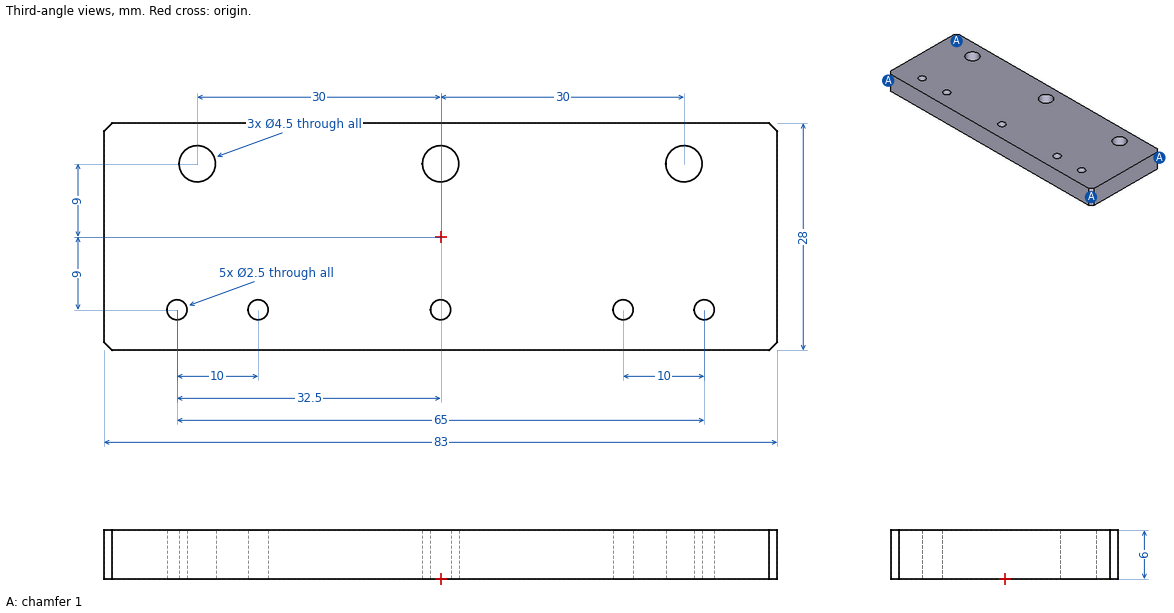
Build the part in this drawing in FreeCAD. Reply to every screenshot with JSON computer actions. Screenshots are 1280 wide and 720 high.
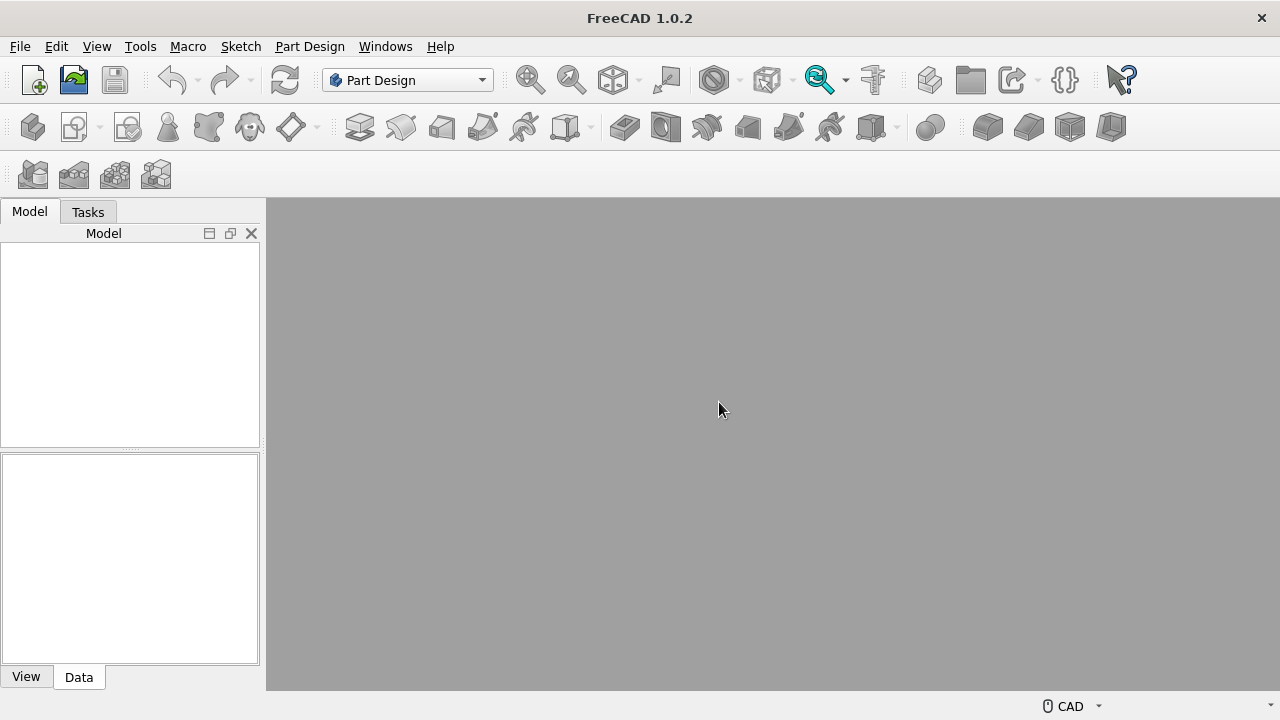
{"action": "left_click", "coordinate": [33, 80]}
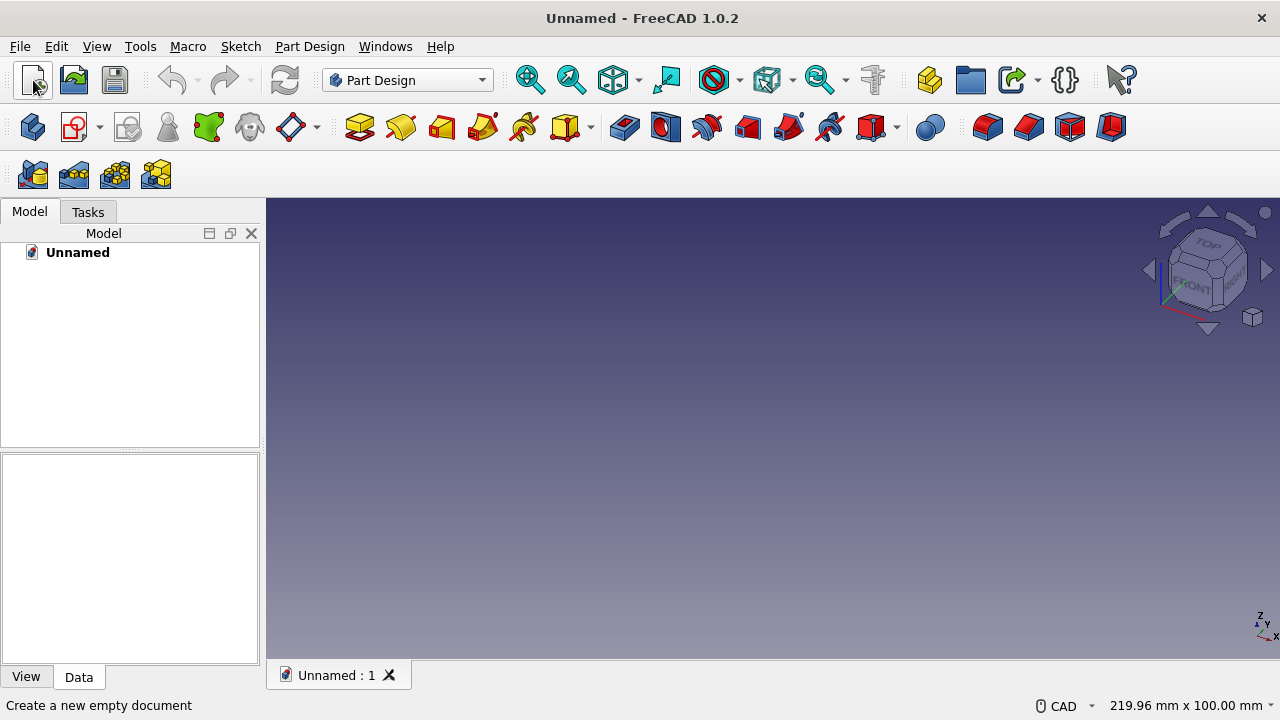
{"action": "left_click", "coordinate": [74, 128]}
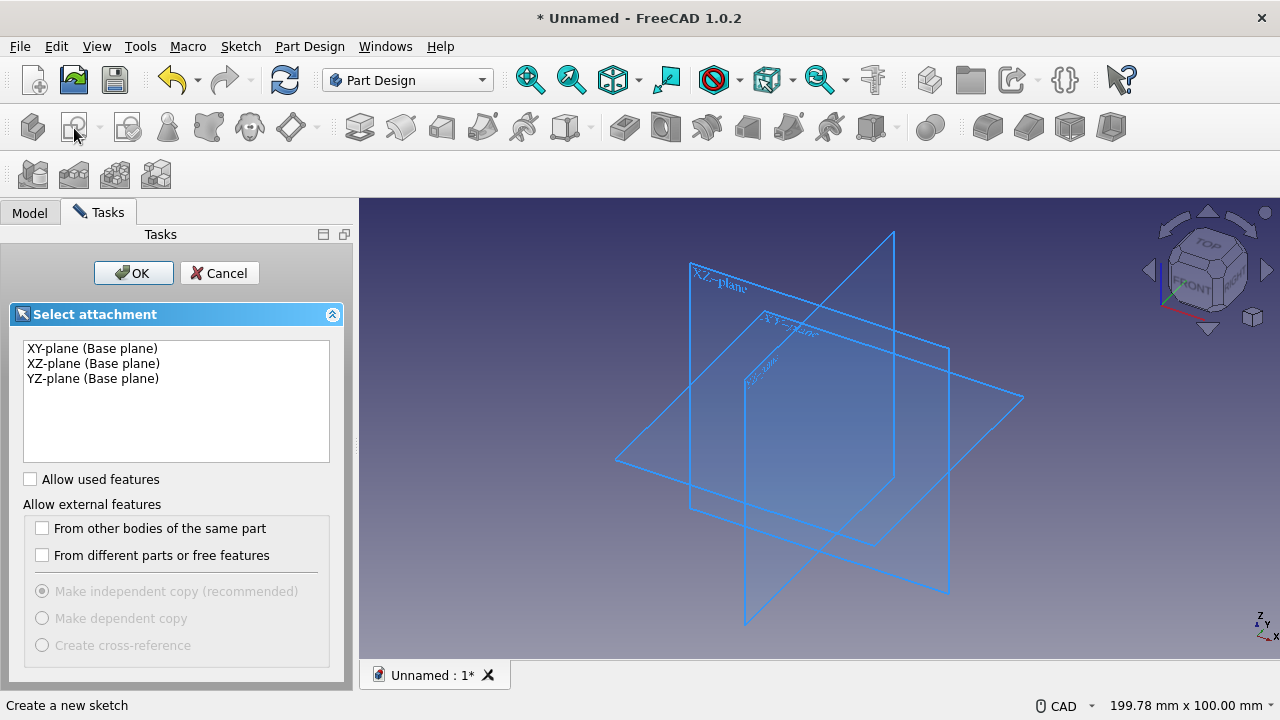
{"action": "left_click", "coordinate": [84, 348]}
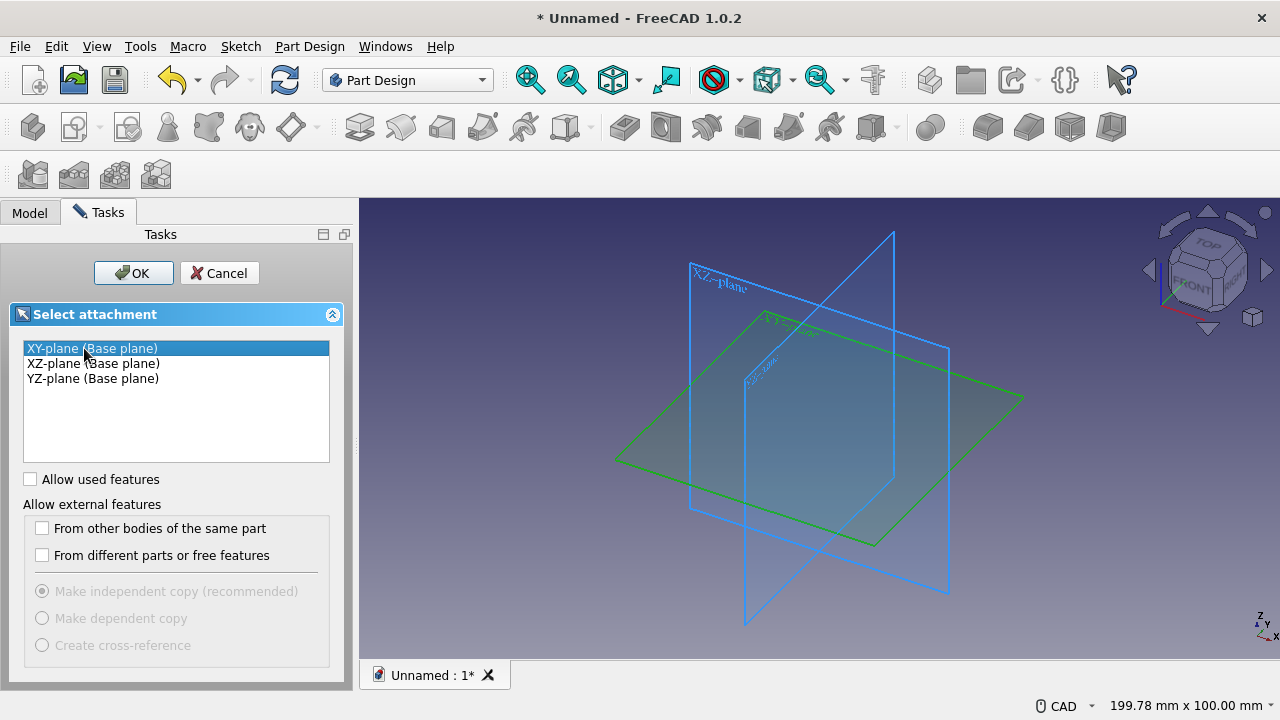
{"action": "left_click", "coordinate": [134, 273]}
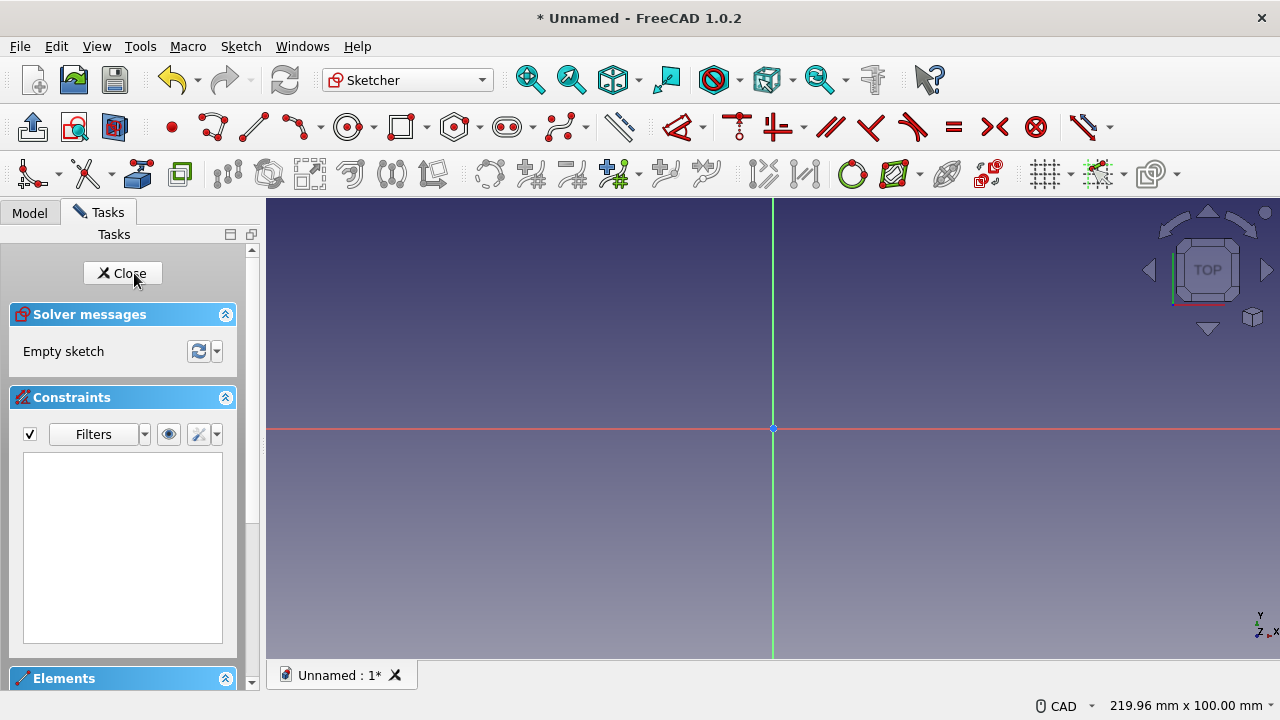
{"action": "scroll", "coordinate": [912, 428], "scroll_direction": "up", "scroll_amount": 2}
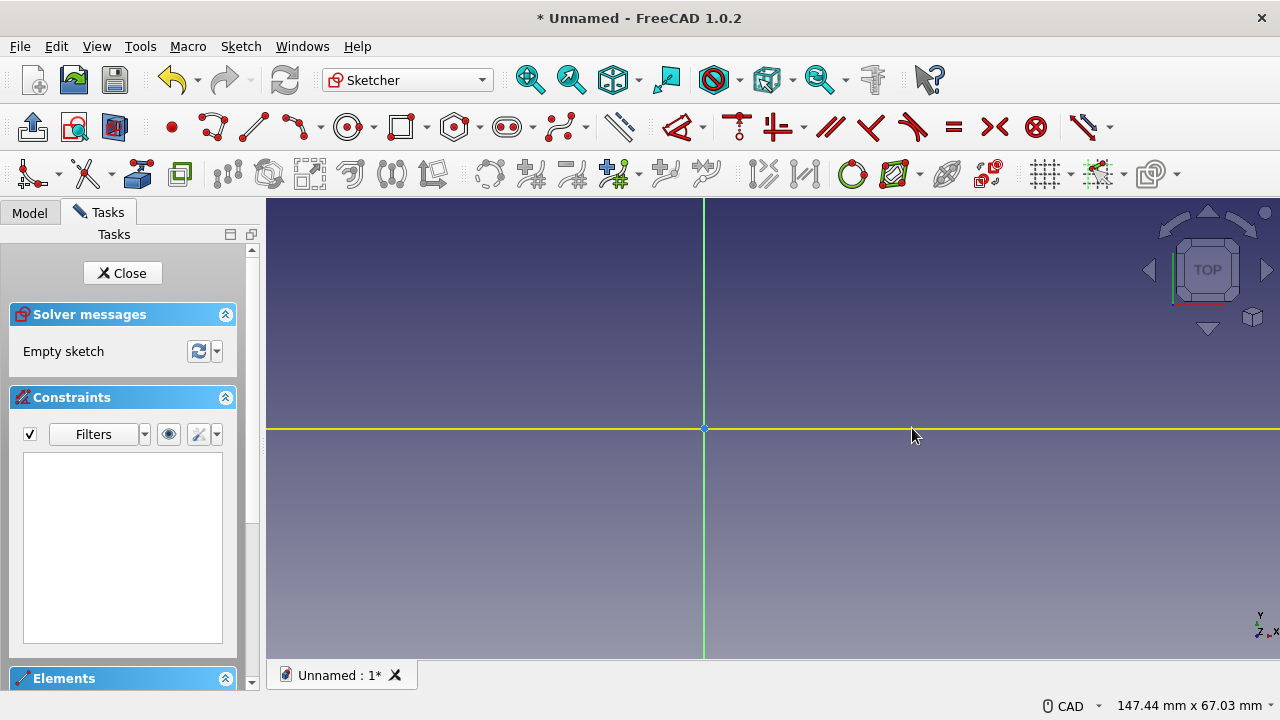
{"action": "key", "text": "g v"}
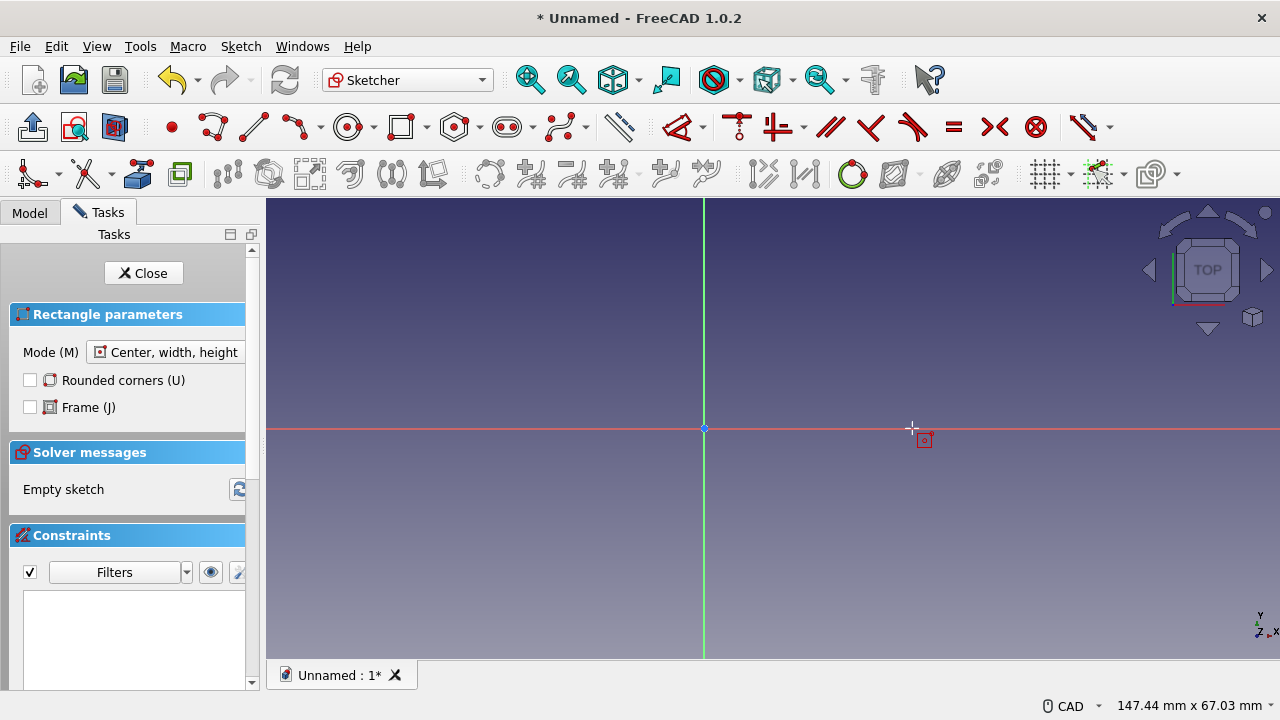
{"action": "left_click", "coordinate": [704, 428]}
{"action": "left_click", "coordinate": [990, 332]}
{"action": "key", "text": "Escape"}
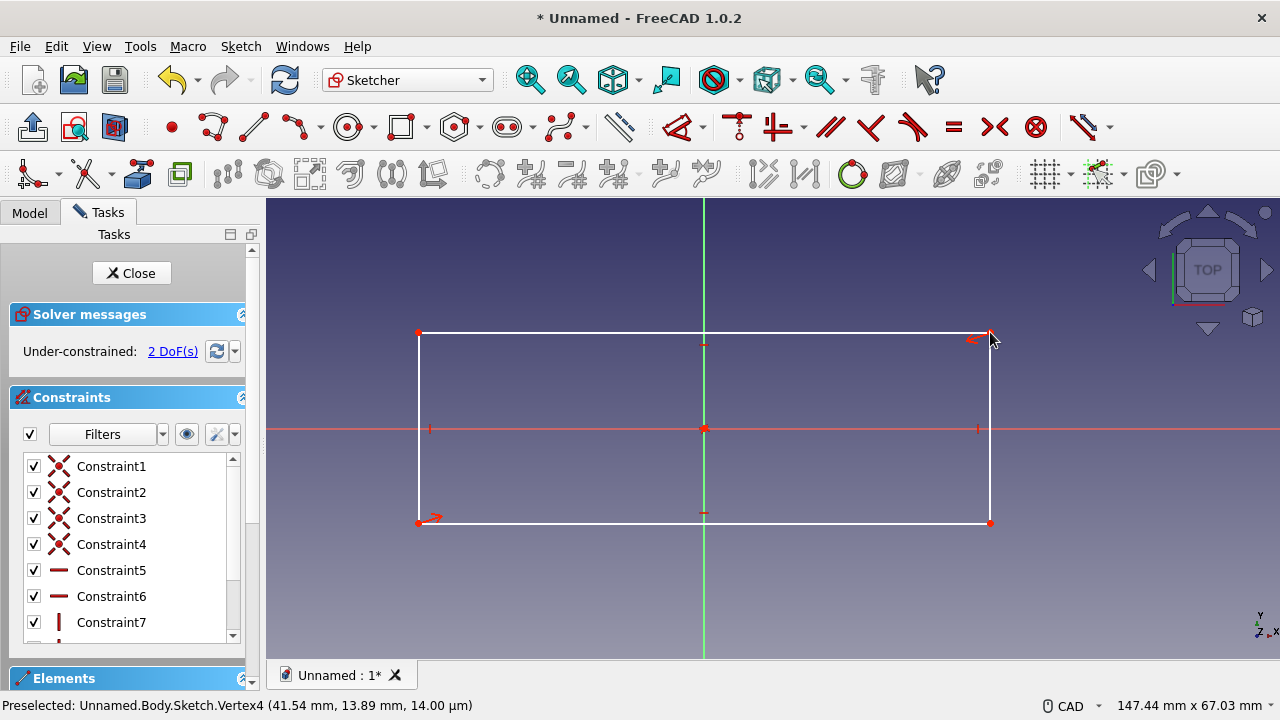
{"action": "left_click", "coordinate": [676, 128]}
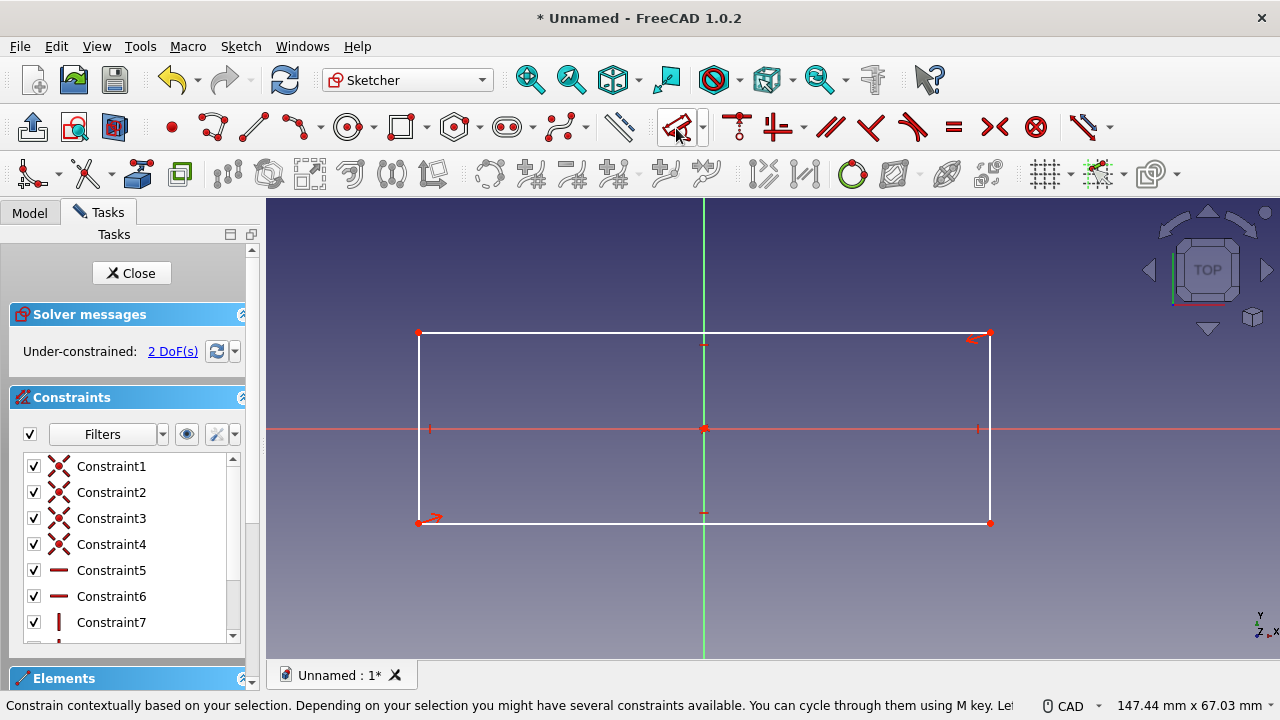
{"action": "left_click", "coordinate": [590, 524]}
{"action": "left_click", "coordinate": [573, 558]}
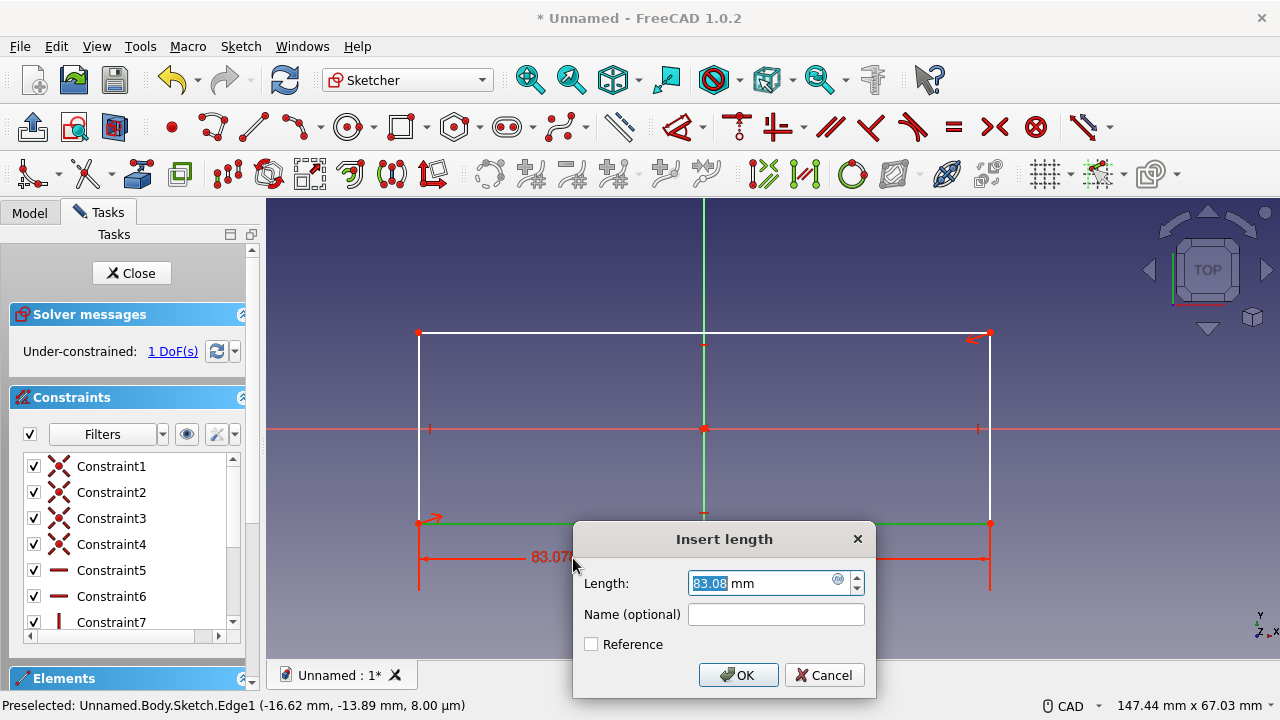
{"action": "type", "text": "83"}
{"action": "key", "text": "Return"}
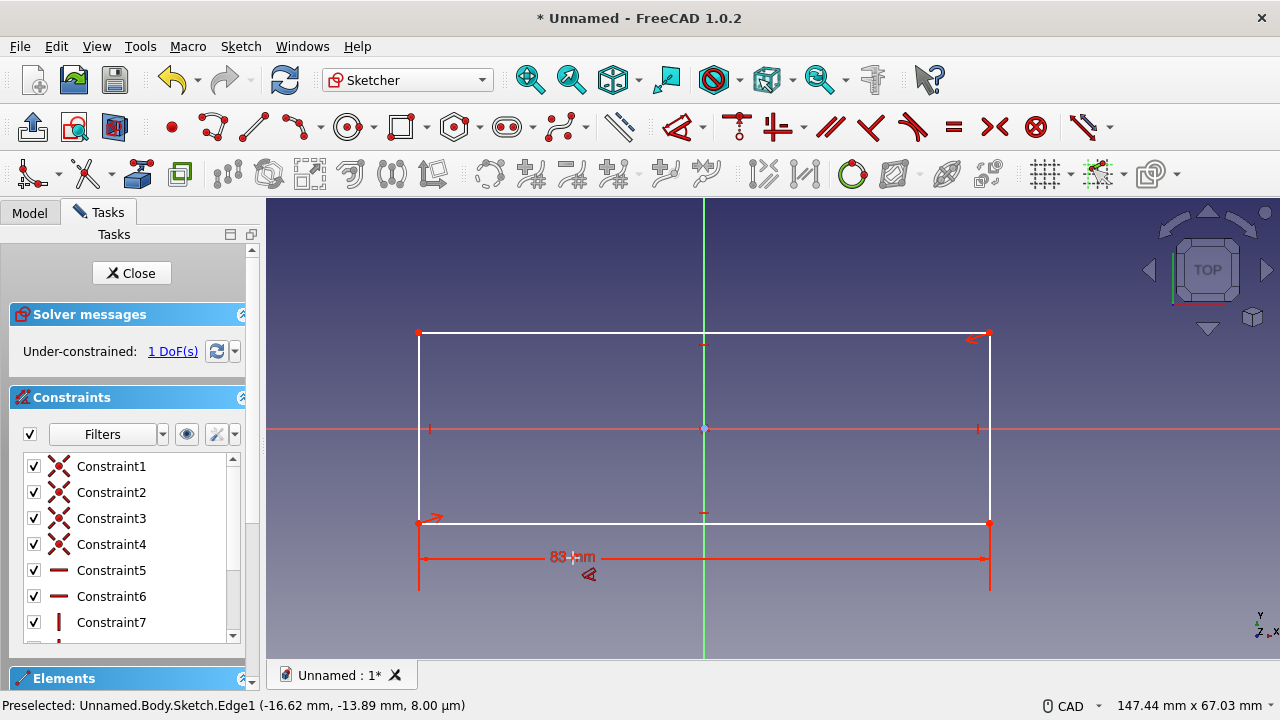
{"action": "left_click", "coordinate": [990, 467]}
{"action": "left_click", "coordinate": [1024, 385]}